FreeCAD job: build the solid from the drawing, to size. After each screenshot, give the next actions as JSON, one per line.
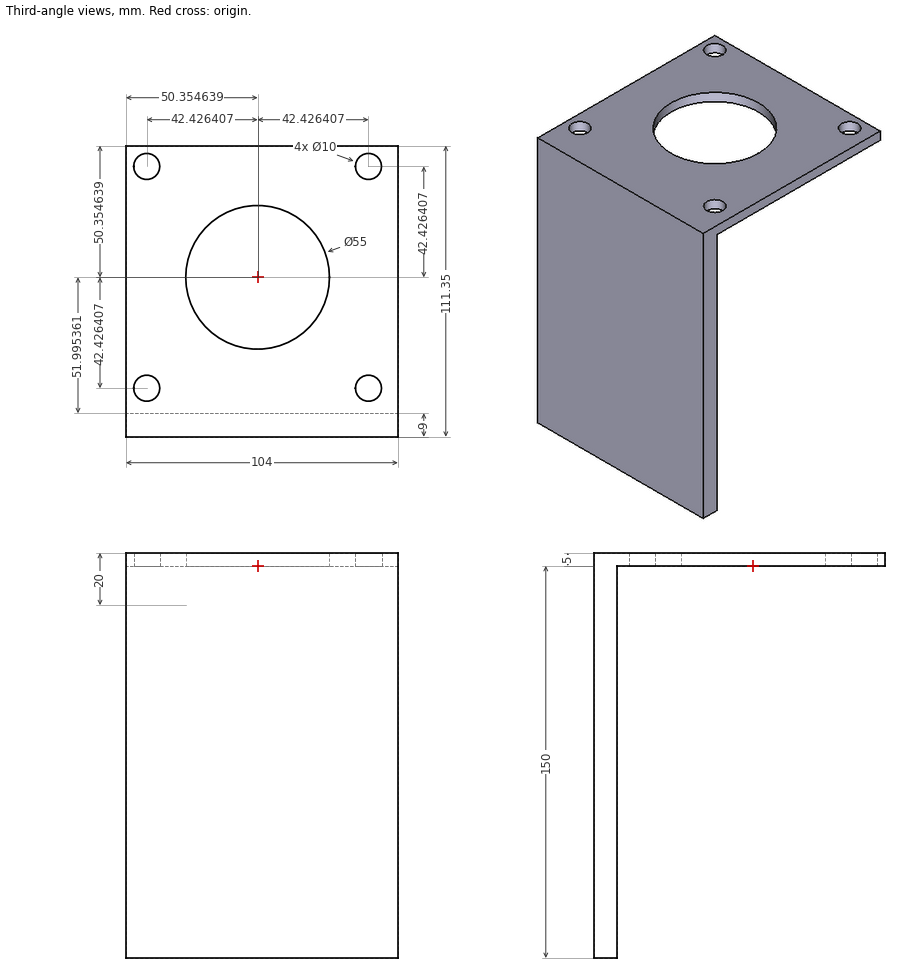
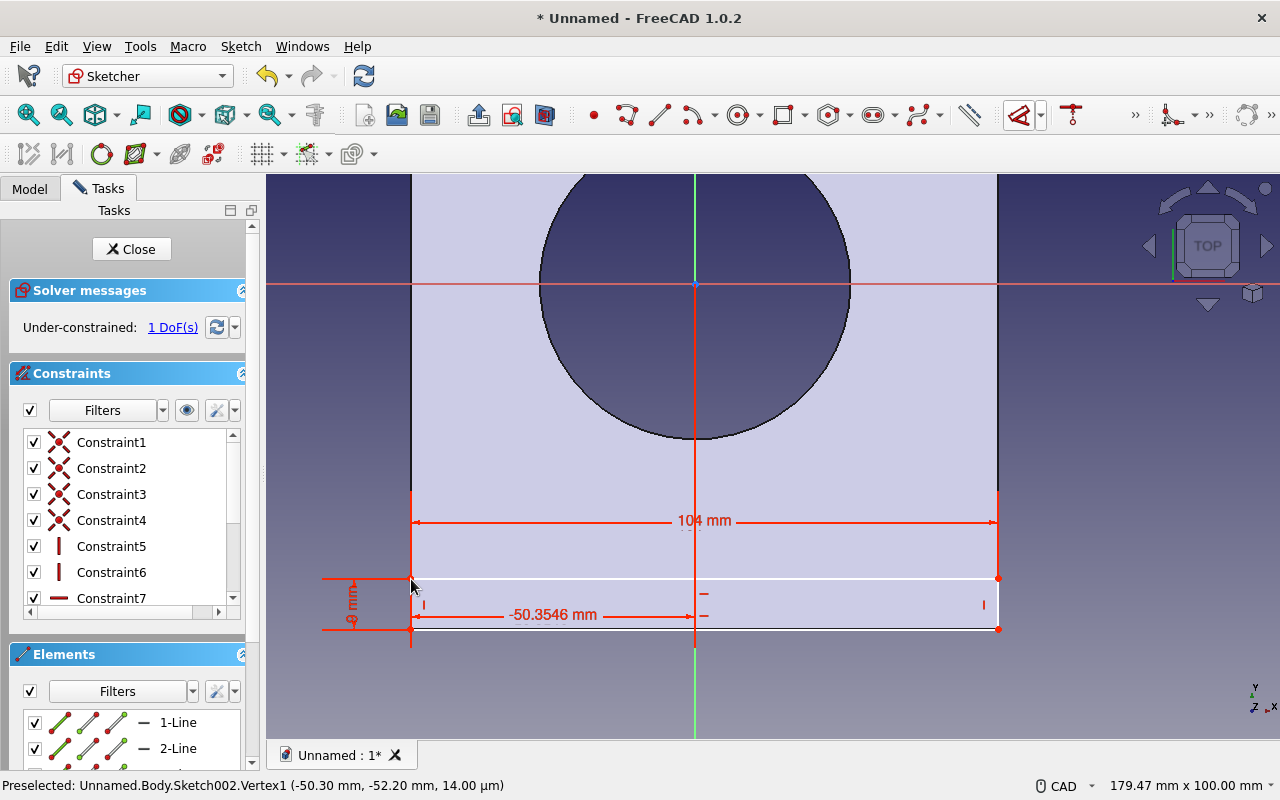
{"action": "left_click", "coordinate": [411, 579]}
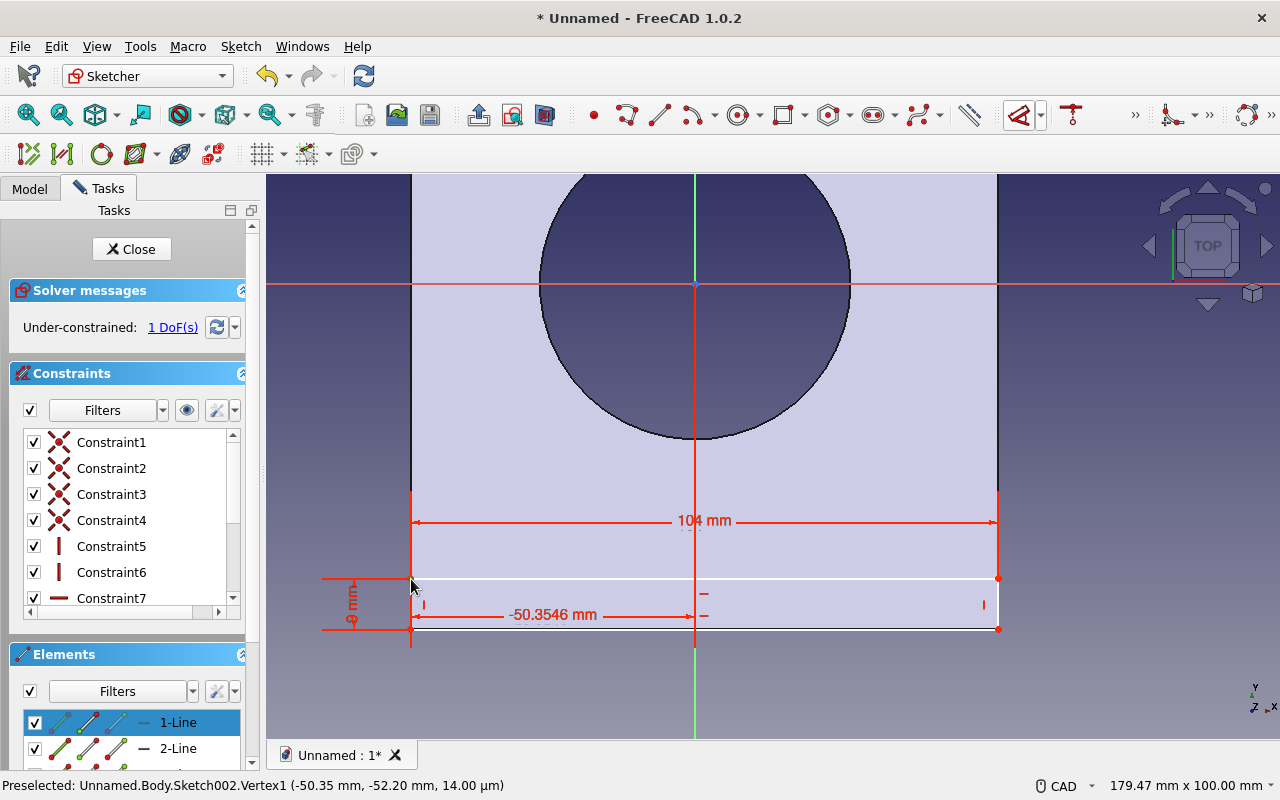
{"action": "left_click", "coordinate": [1040, 116]}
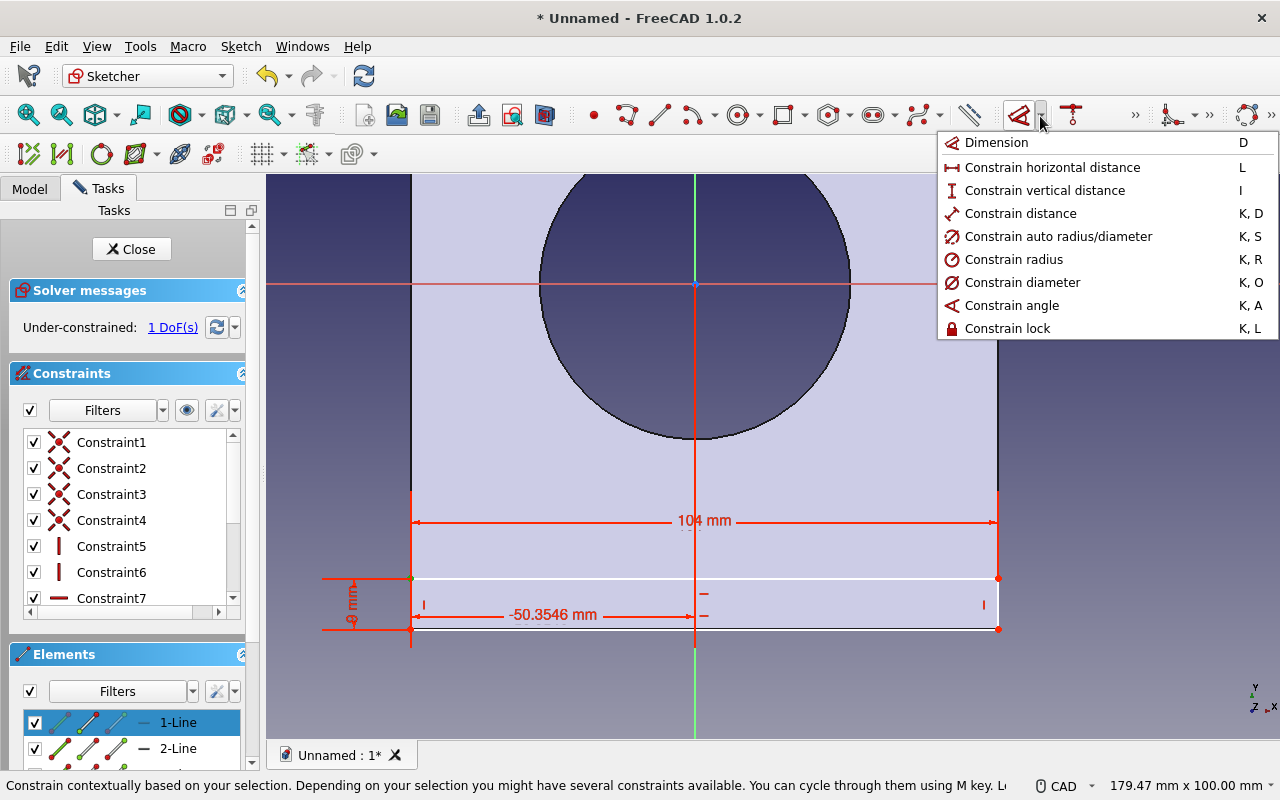
{"action": "left_click", "coordinate": [1108, 190]}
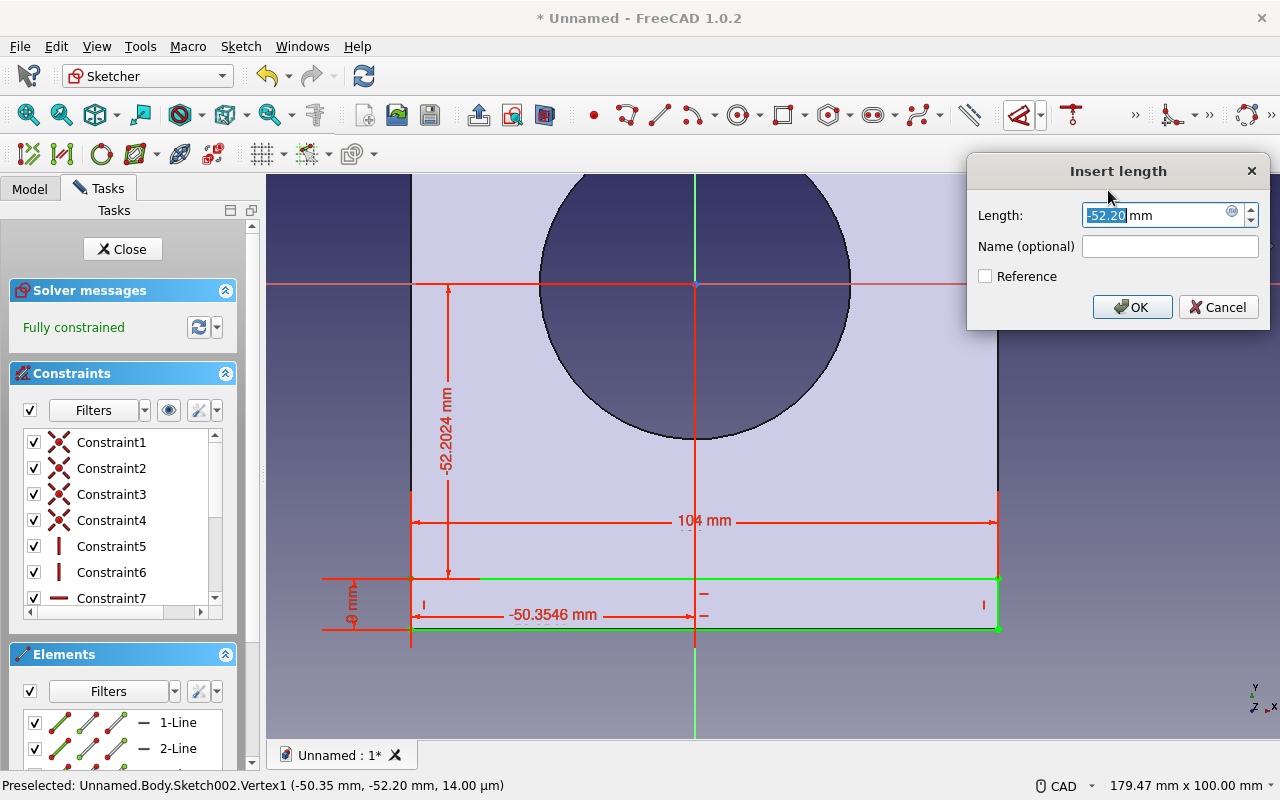
{"action": "type", "text": "-51.995361"}
{"action": "key", "text": "Return"}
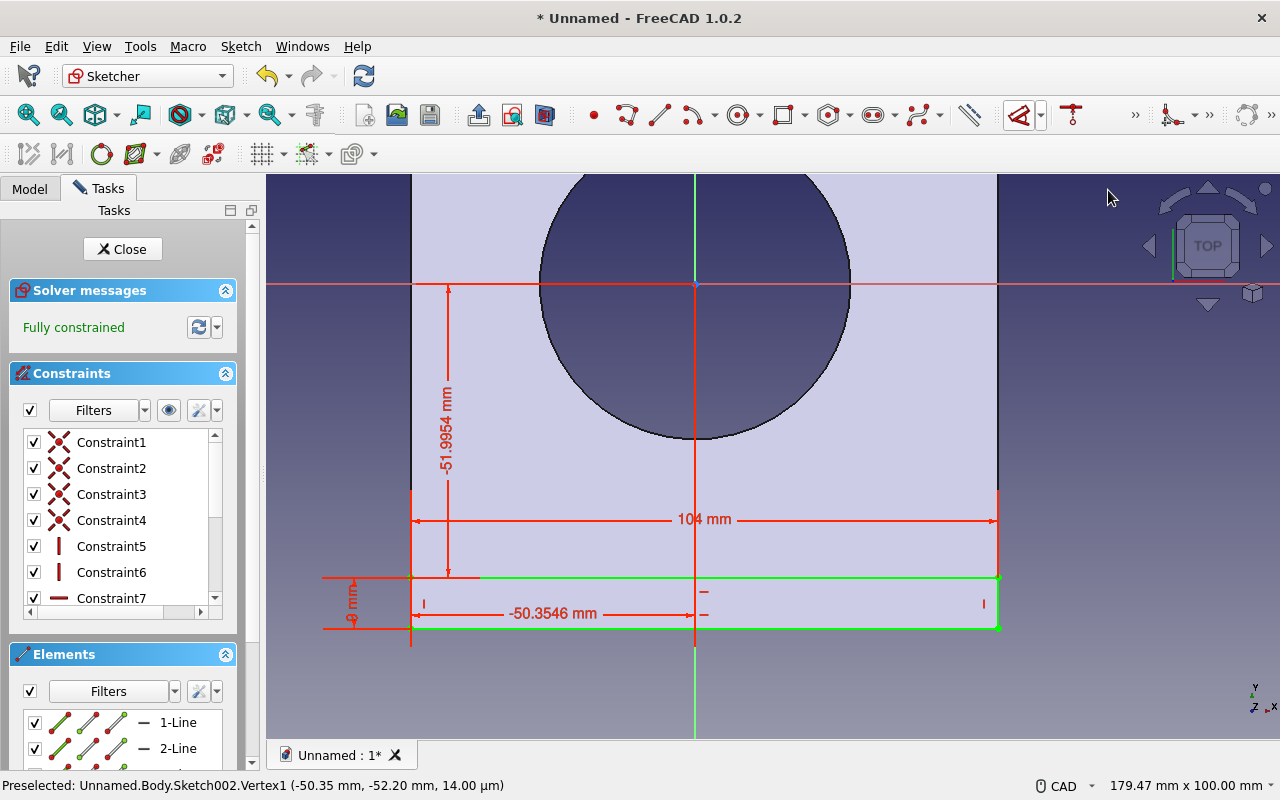
{"action": "left_click", "coordinate": [123, 249]}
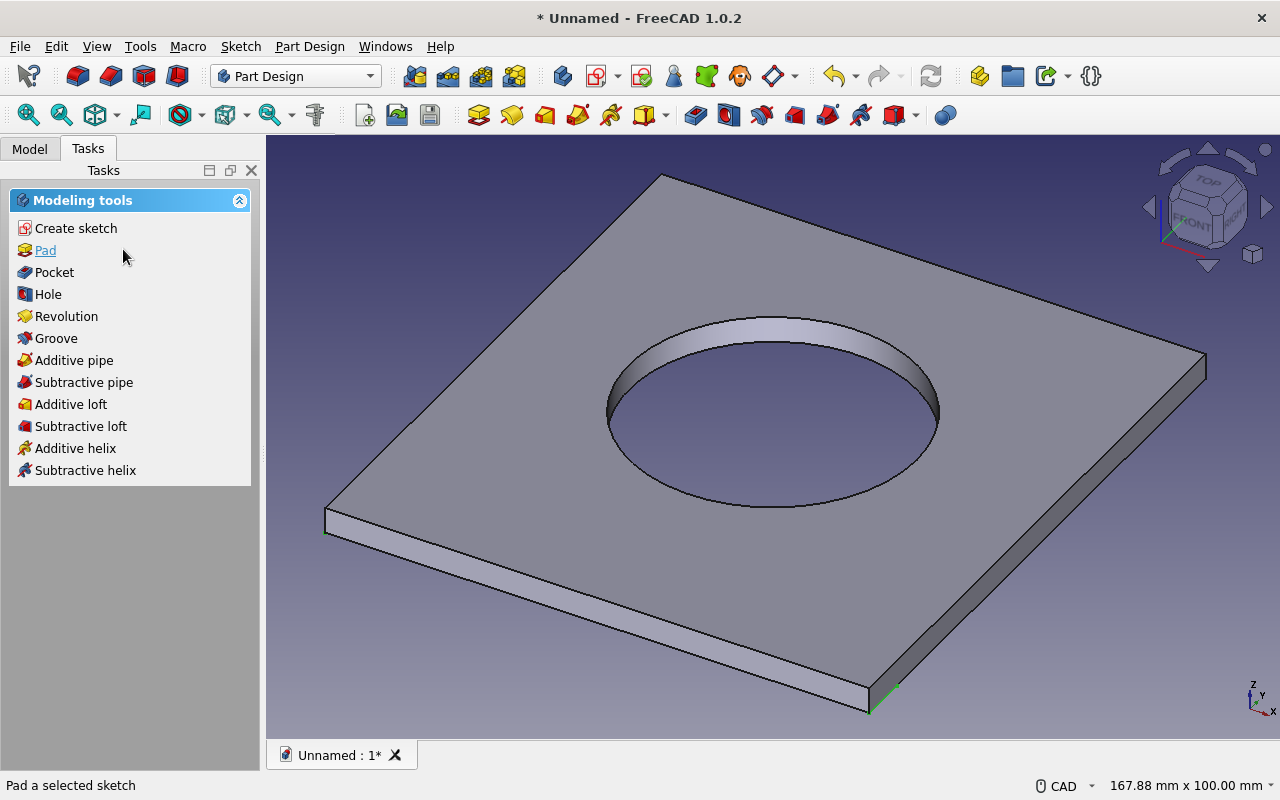
{"action": "left_click", "coordinate": [479, 116]}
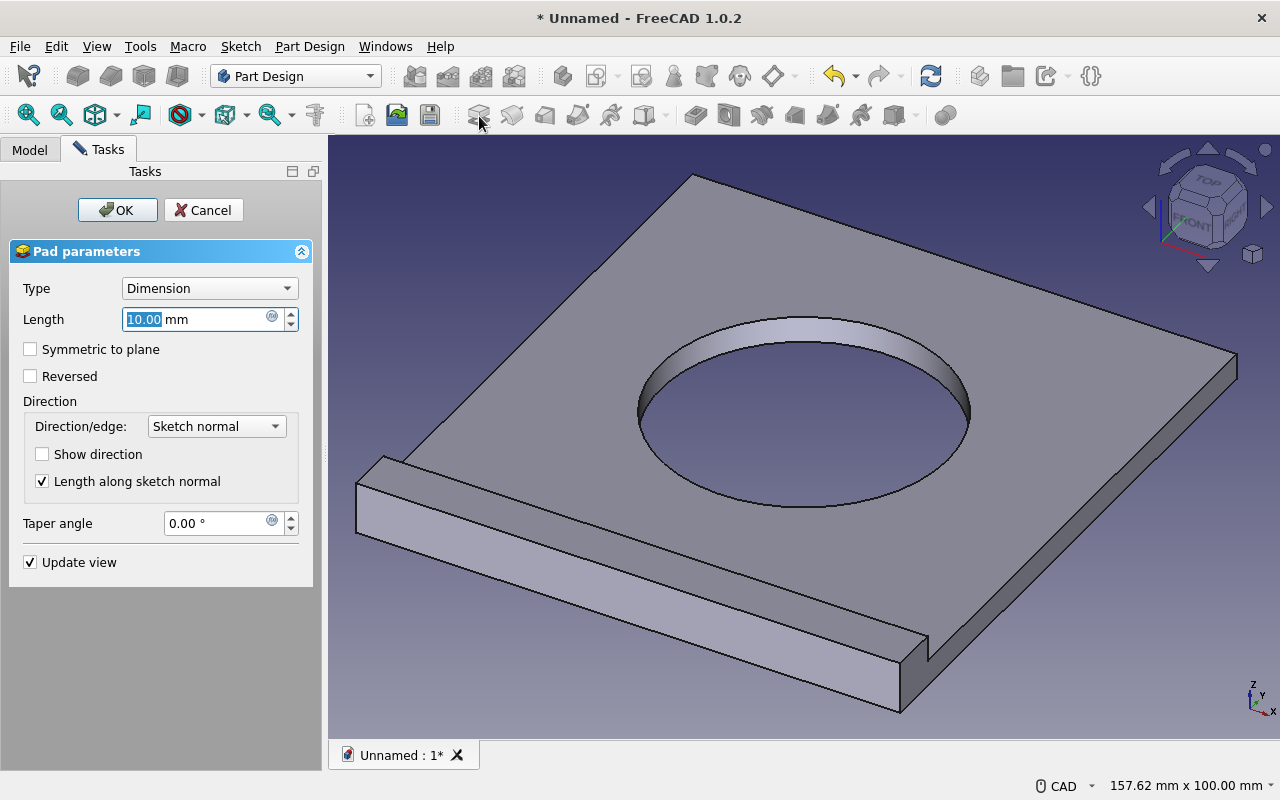
{"action": "type", "text": "150"}
{"action": "key", "text": "Tab"}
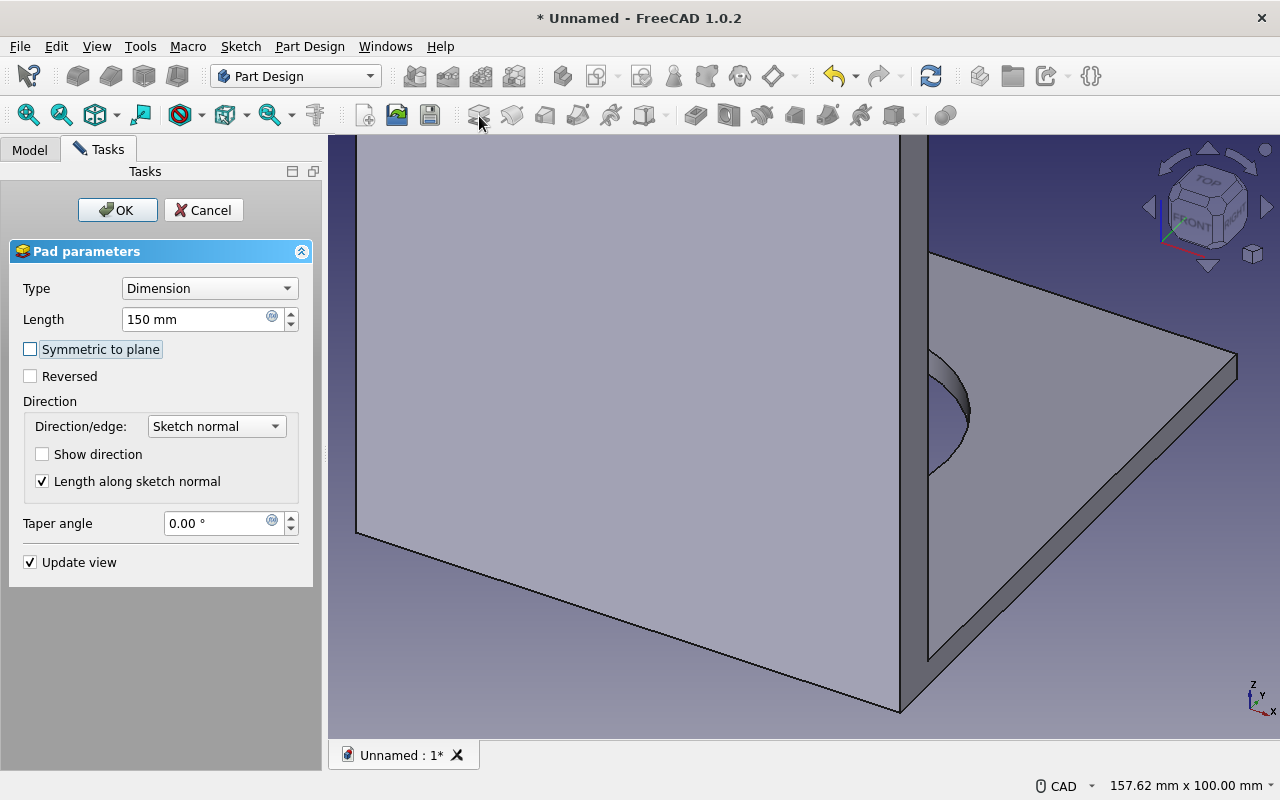
{"action": "left_click", "coordinate": [31, 376]}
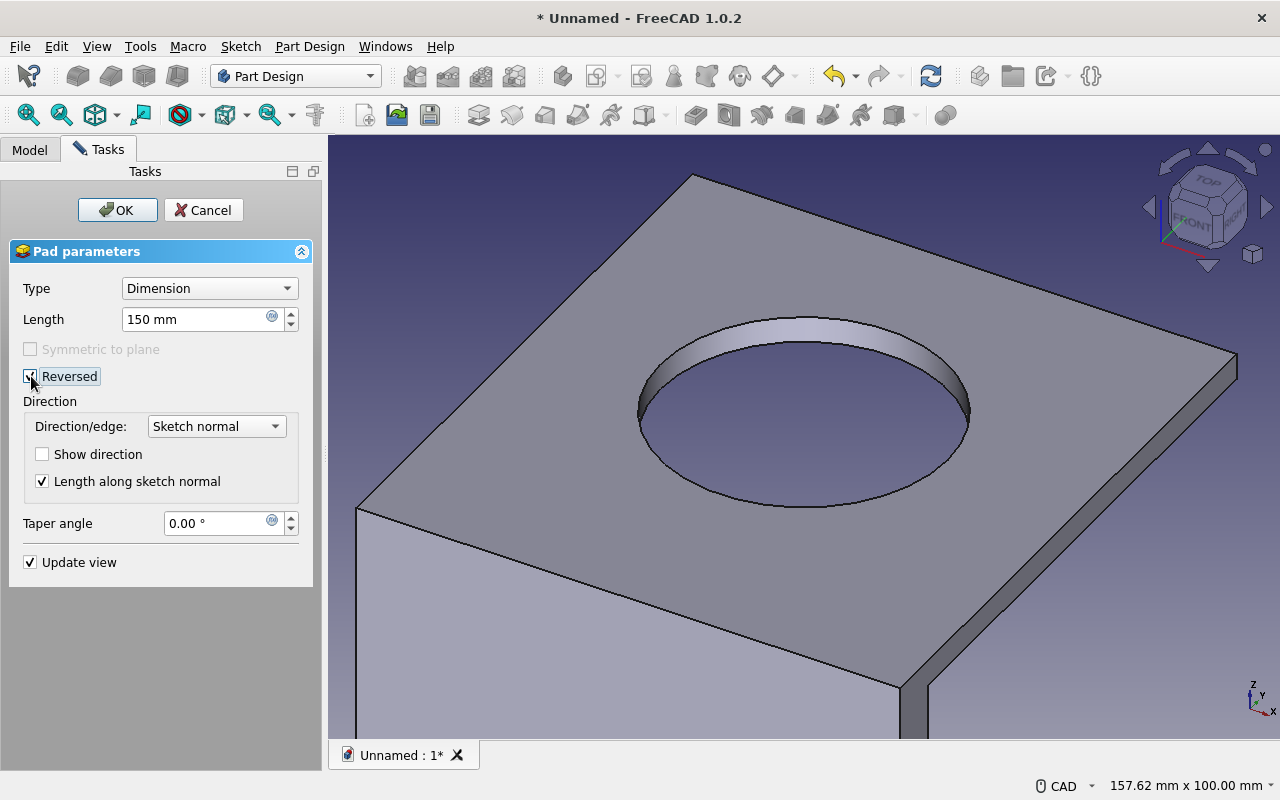
{"action": "left_click", "coordinate": [118, 210]}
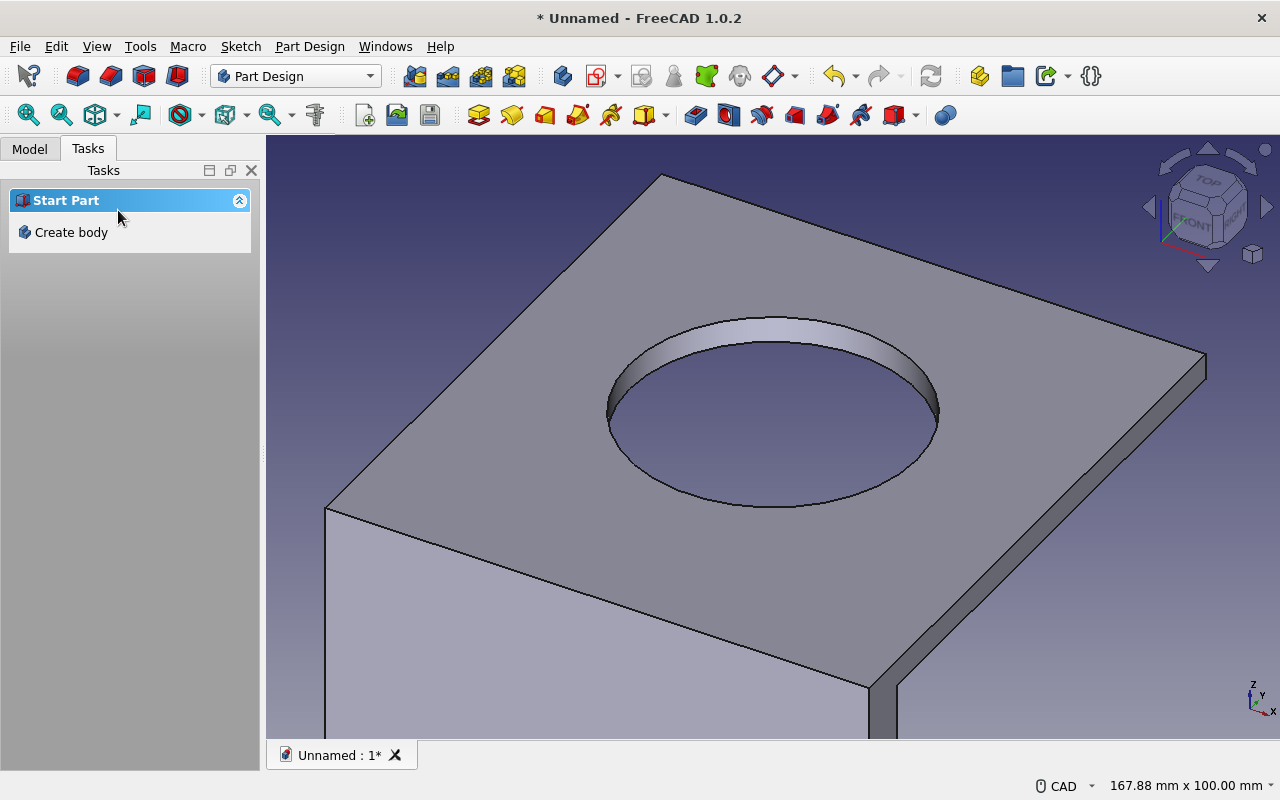
{"action": "key", "text": "v f"}